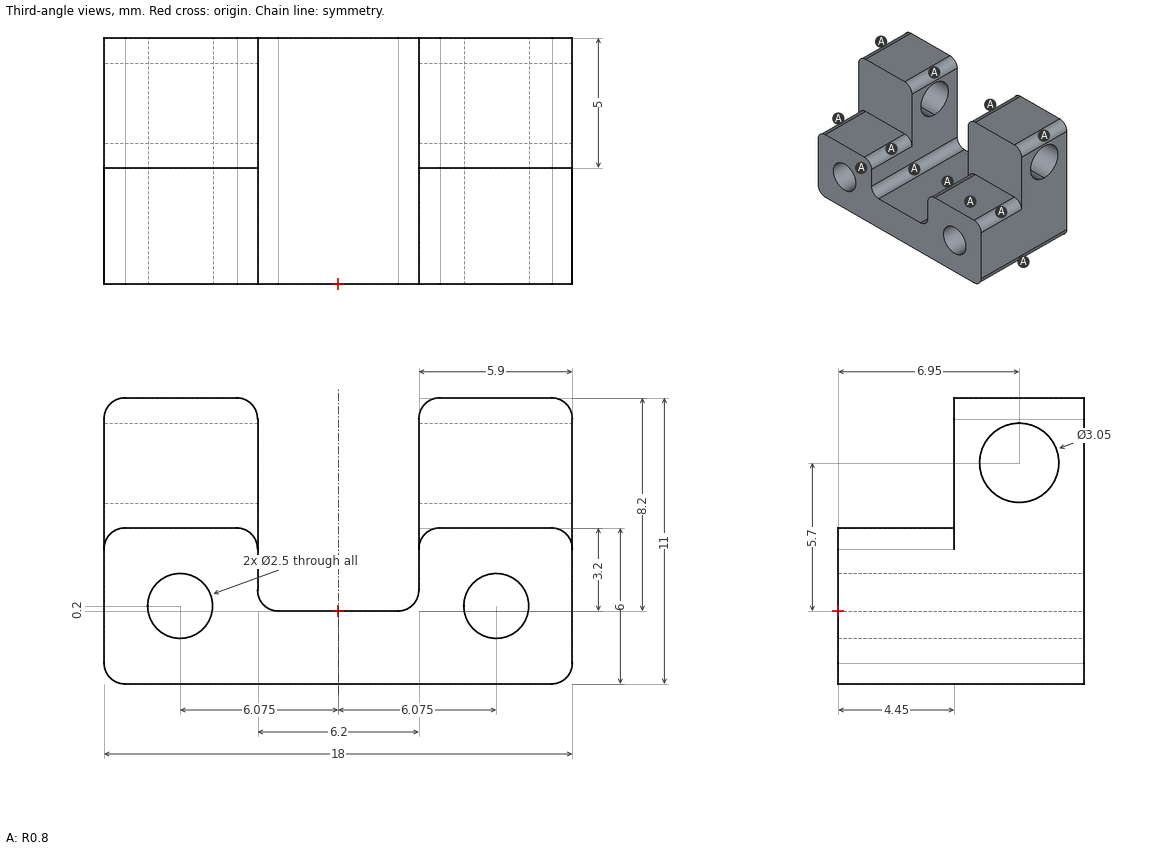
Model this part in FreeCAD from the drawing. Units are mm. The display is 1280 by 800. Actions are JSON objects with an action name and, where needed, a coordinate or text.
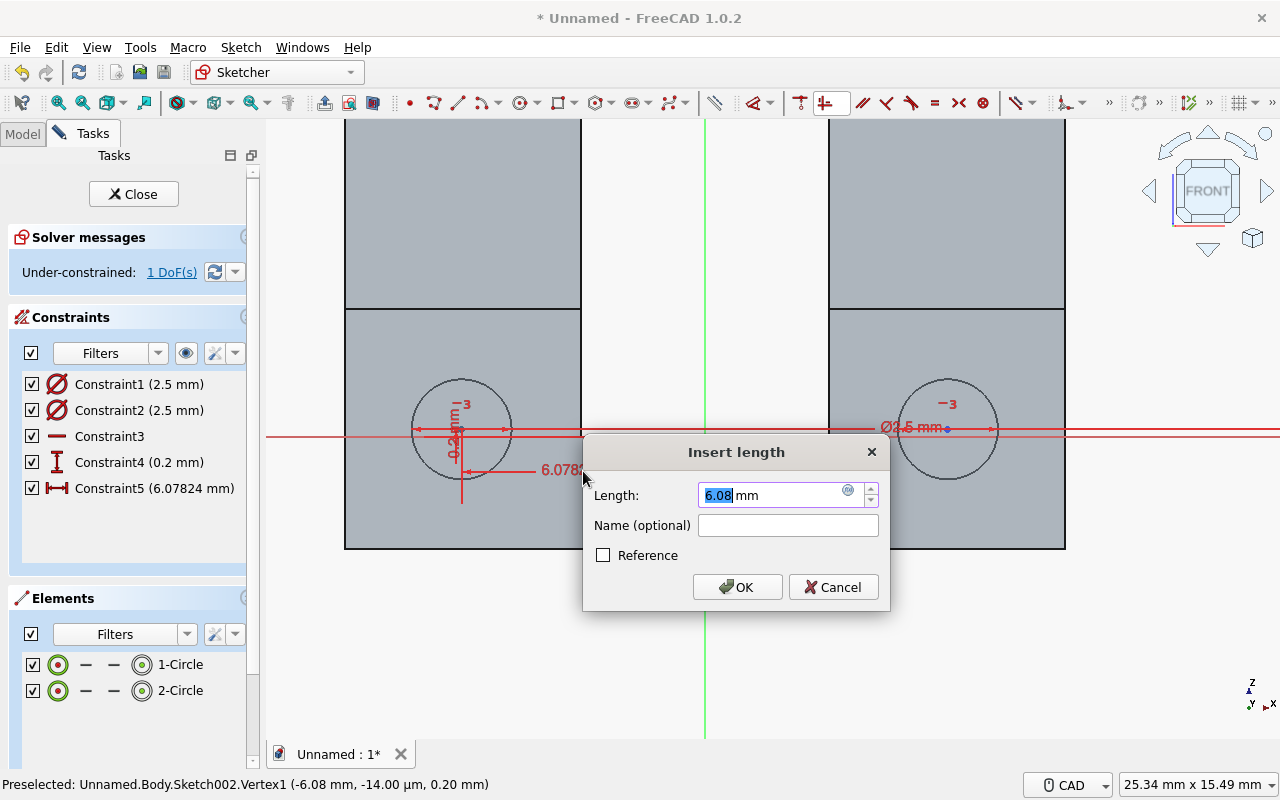
{"action": "type", "text": "6.075"}
{"action": "key", "text": "Return"}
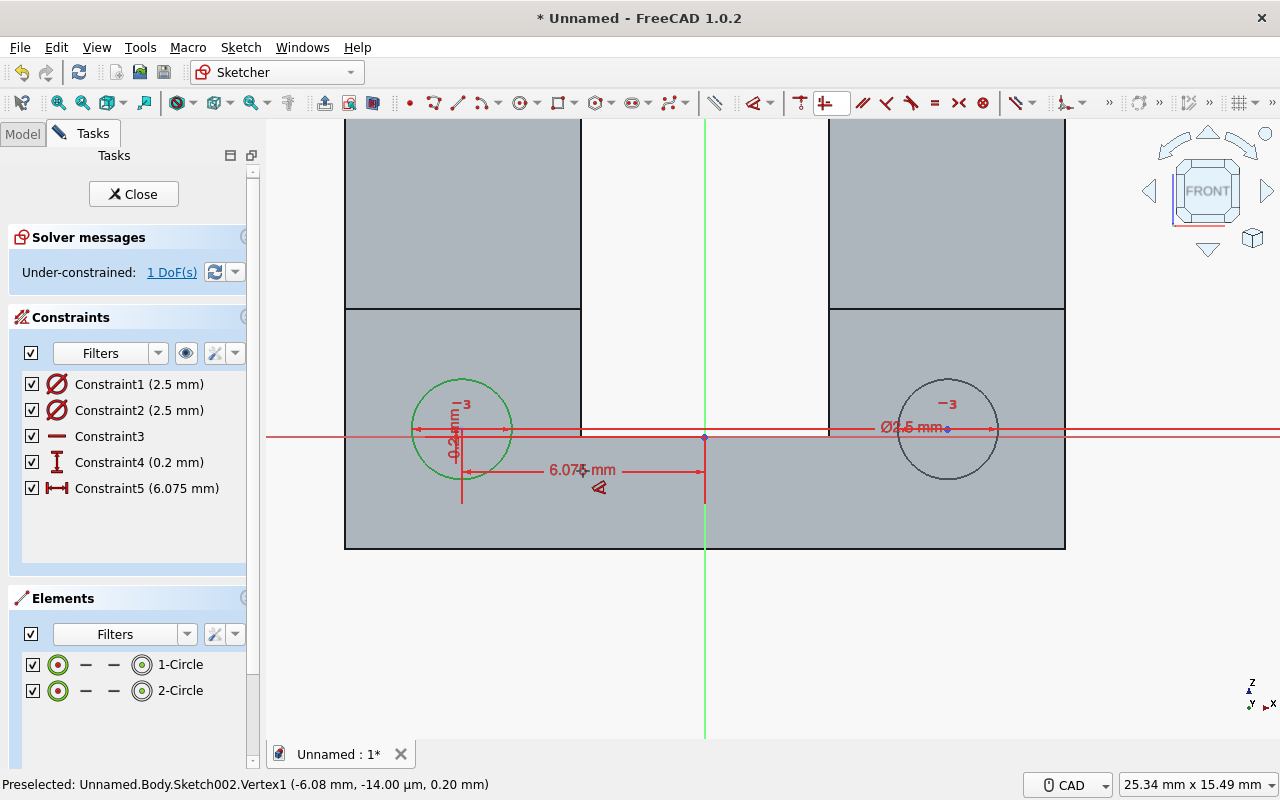
{"action": "left_click", "coordinate": [948, 429]}
{"action": "left_click", "coordinate": [826, 471]}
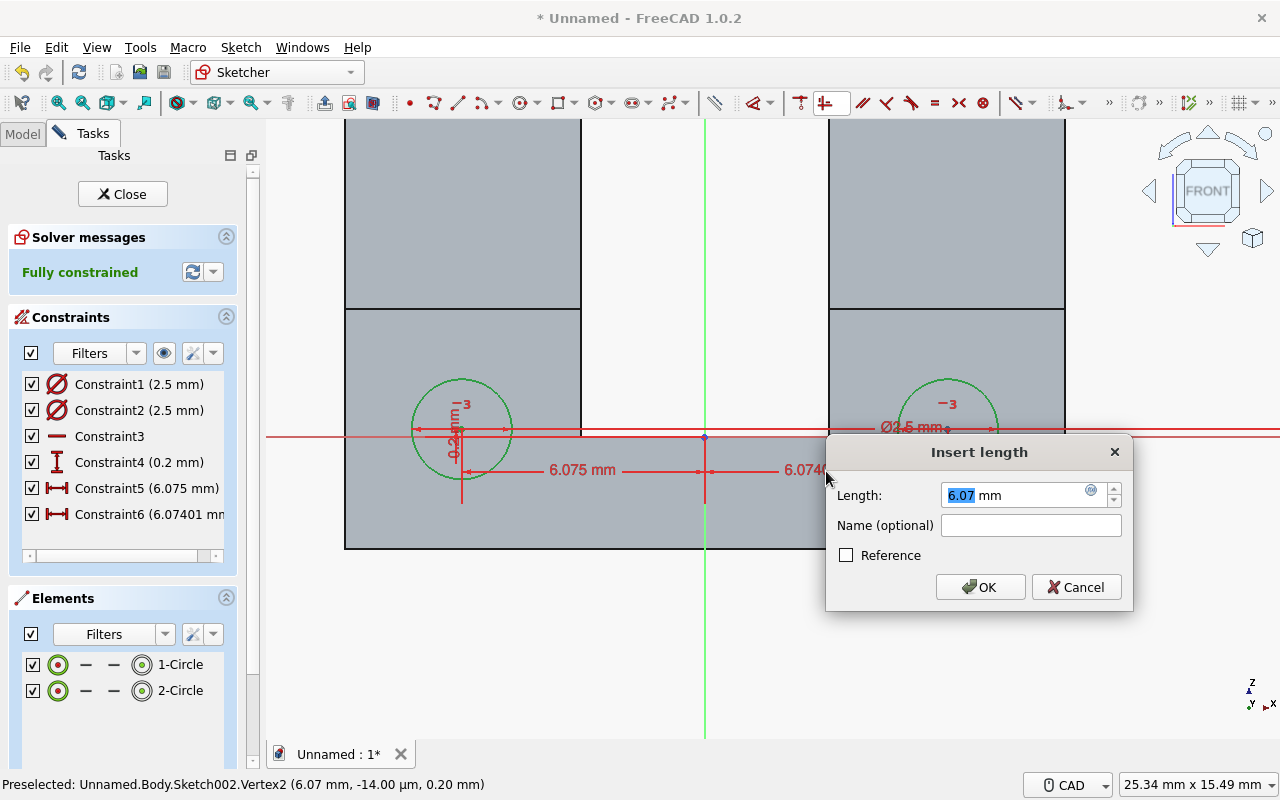
{"action": "type", "text": "6.075"}
{"action": "key", "text": "Return"}
{"action": "key", "text": "Escape"}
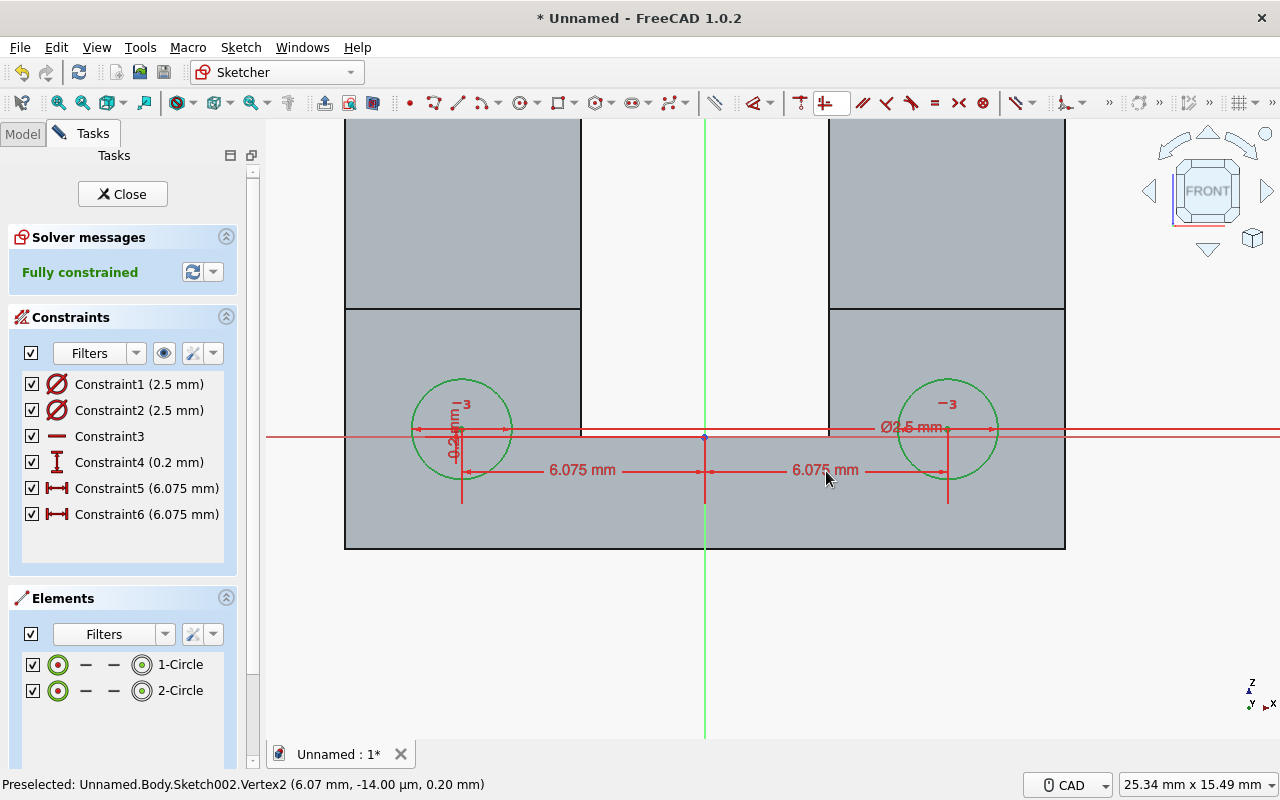
{"action": "left_click", "coordinate": [123, 194]}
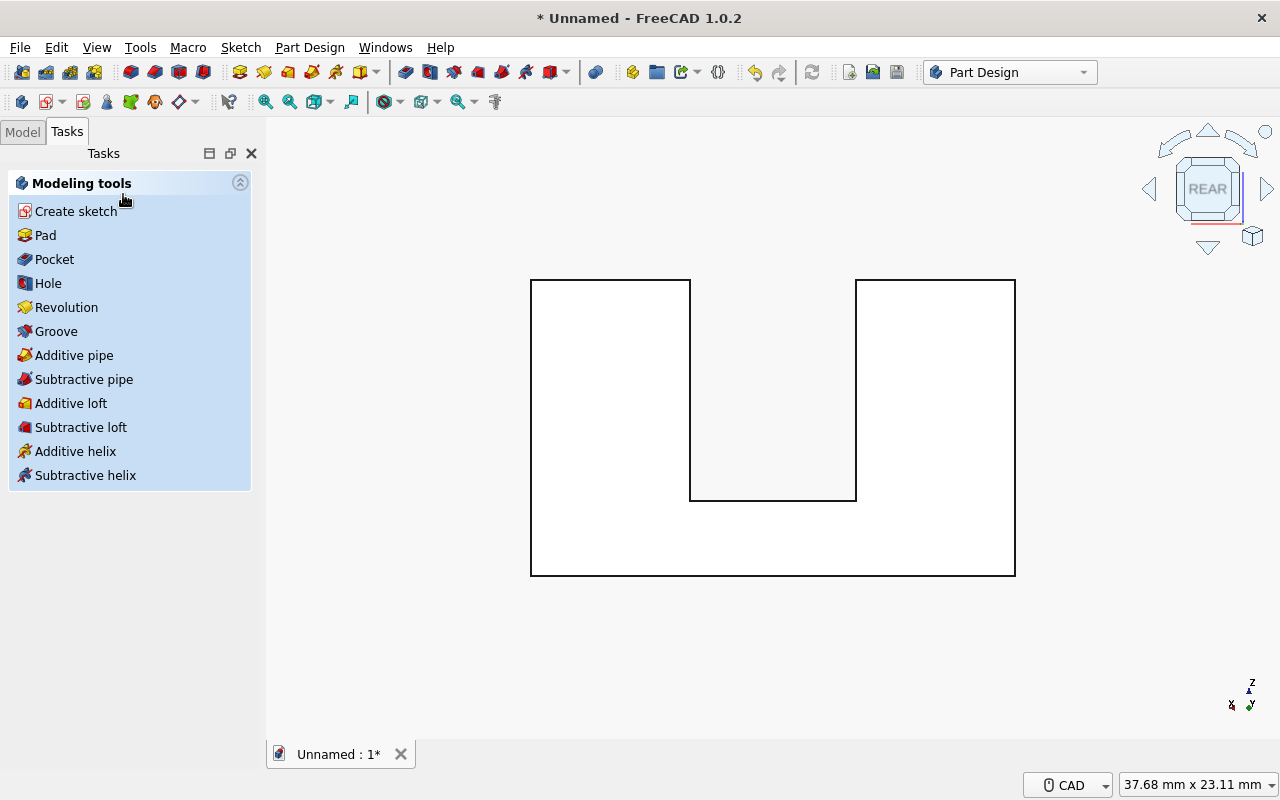
{"action": "left_click", "coordinate": [430, 72]}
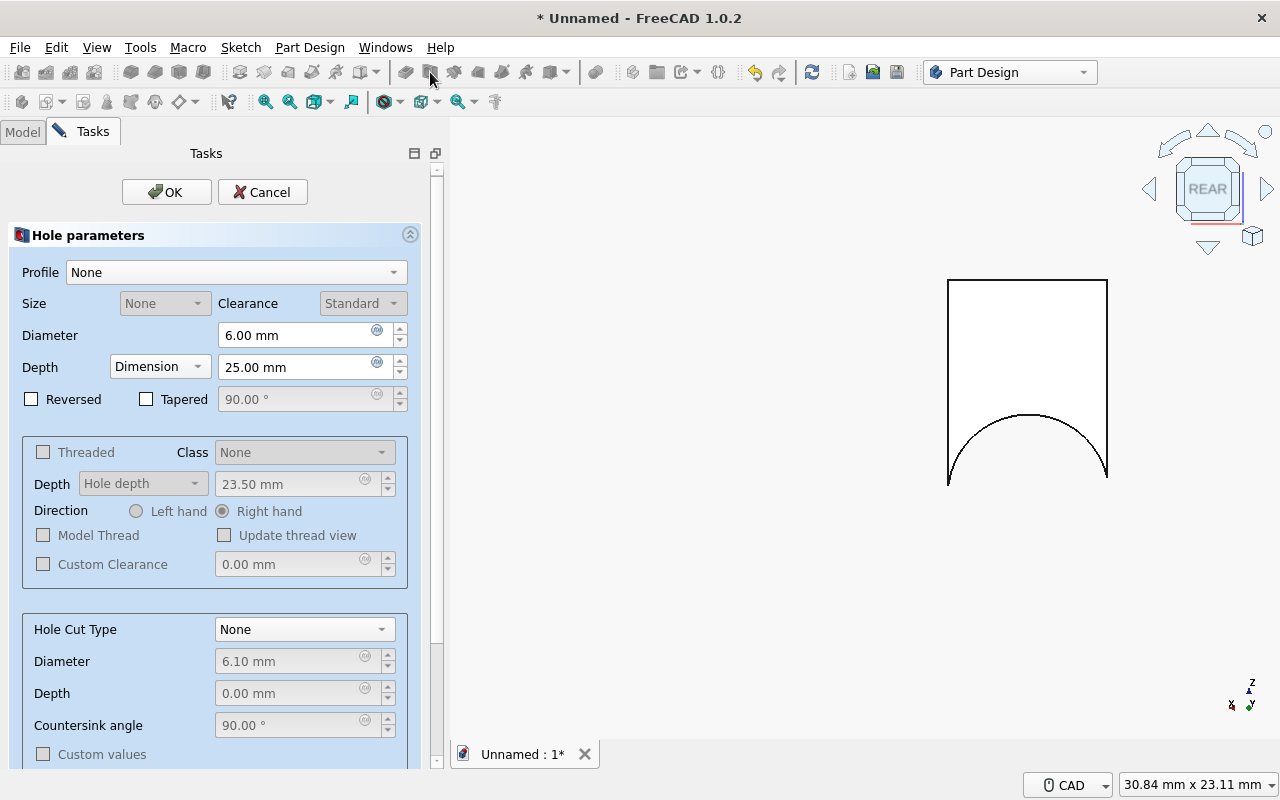
{"action": "triple_click", "coordinate": [305, 335]}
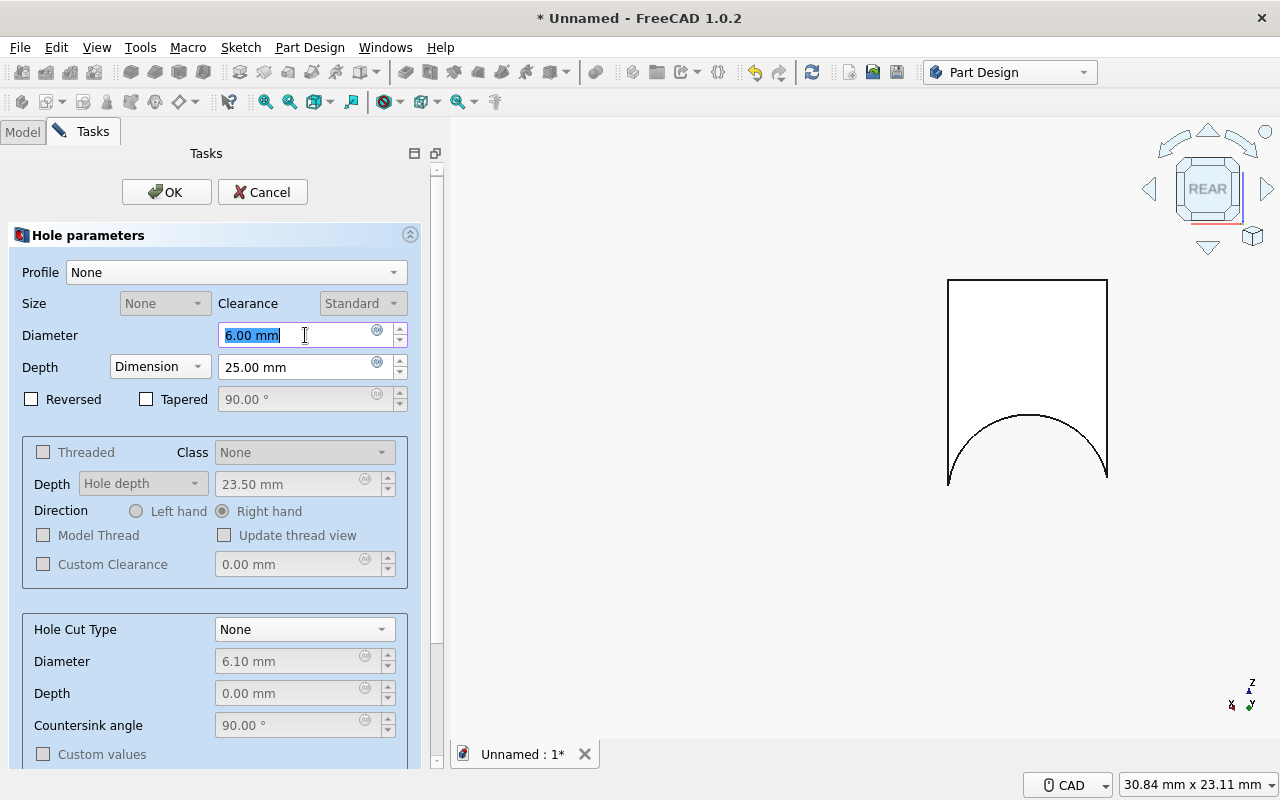
{"action": "type", "text": "2.5"}
{"action": "key", "text": "Tab"}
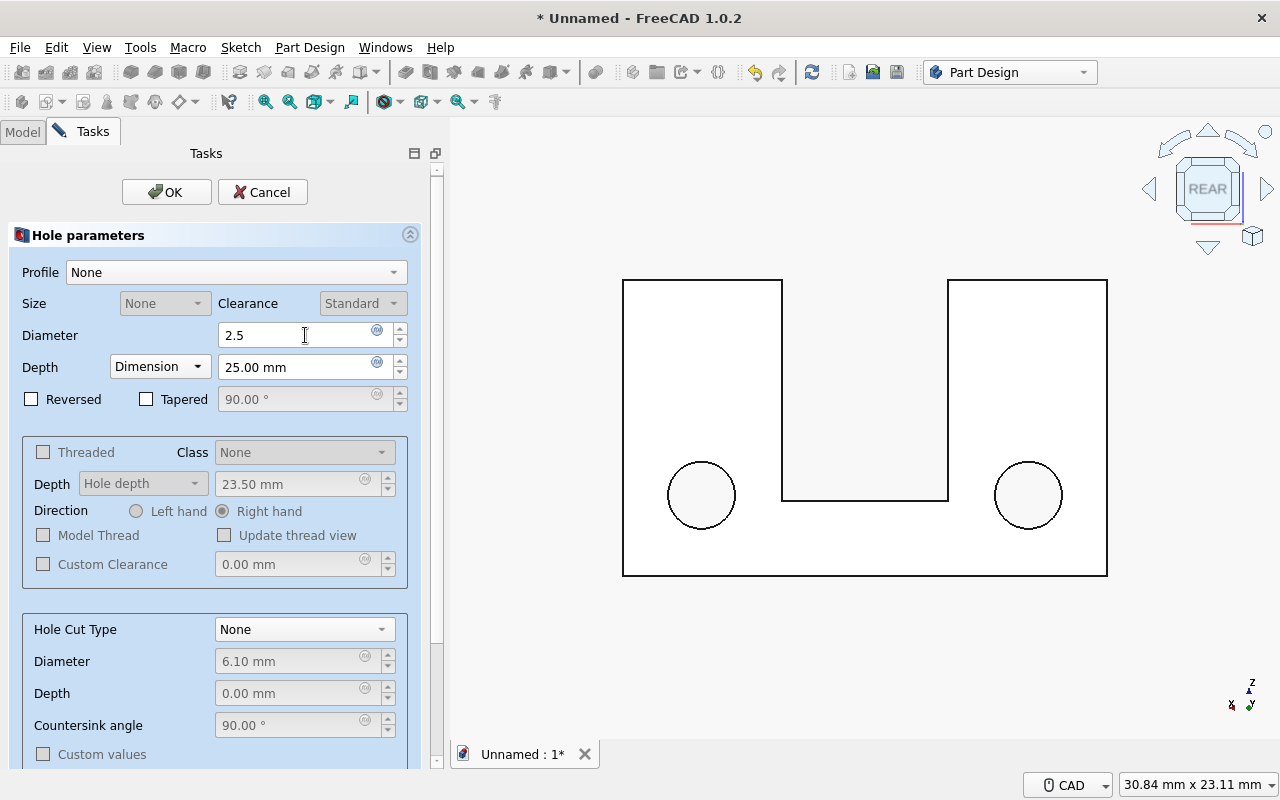
{"action": "left_click", "coordinate": [161, 366]}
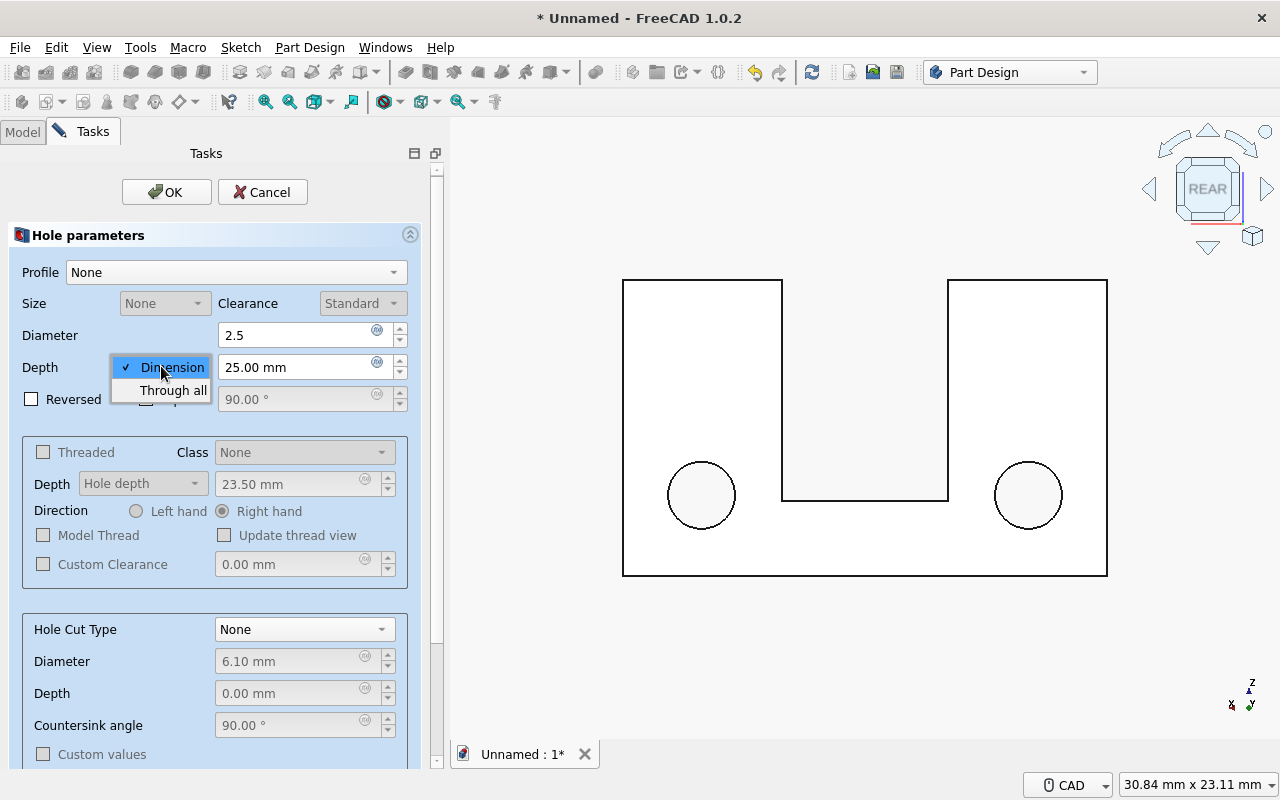
{"action": "left_click", "coordinate": [160, 390]}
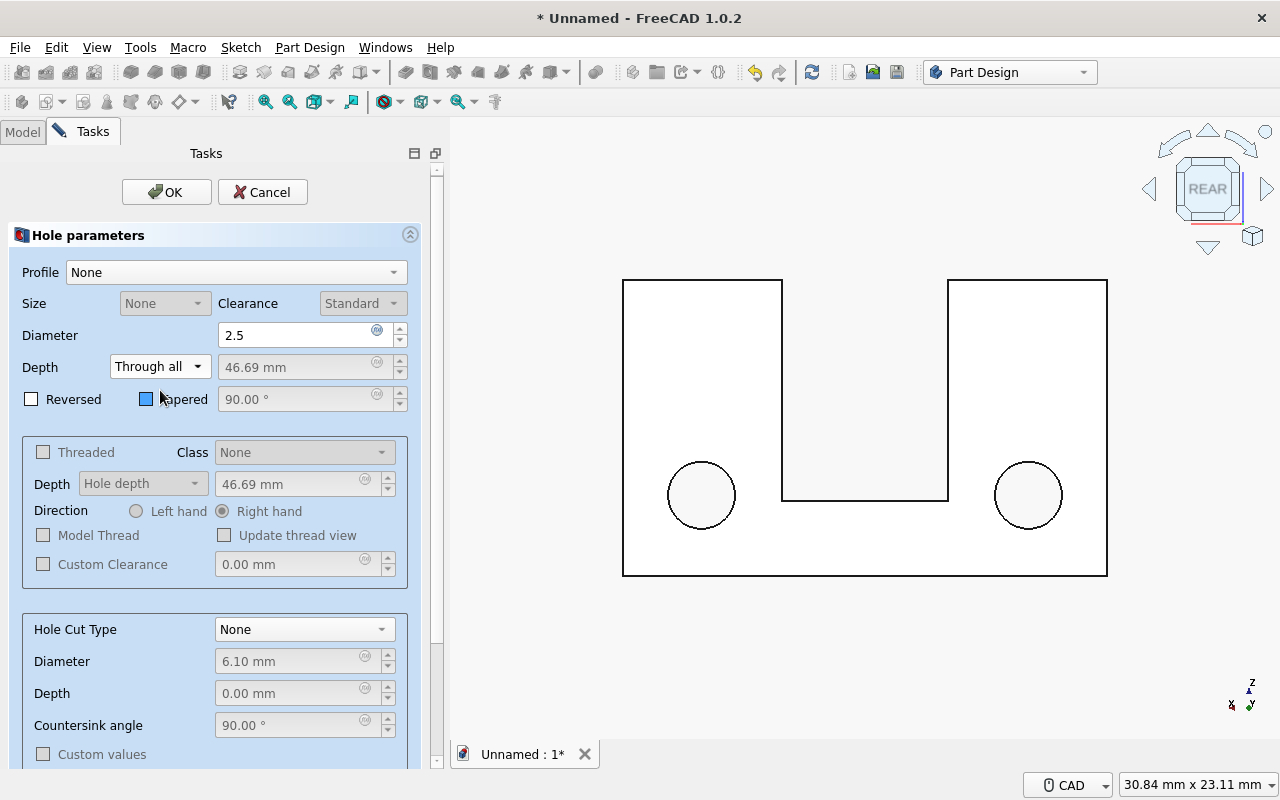
{"action": "left_click", "coordinate": [167, 192]}